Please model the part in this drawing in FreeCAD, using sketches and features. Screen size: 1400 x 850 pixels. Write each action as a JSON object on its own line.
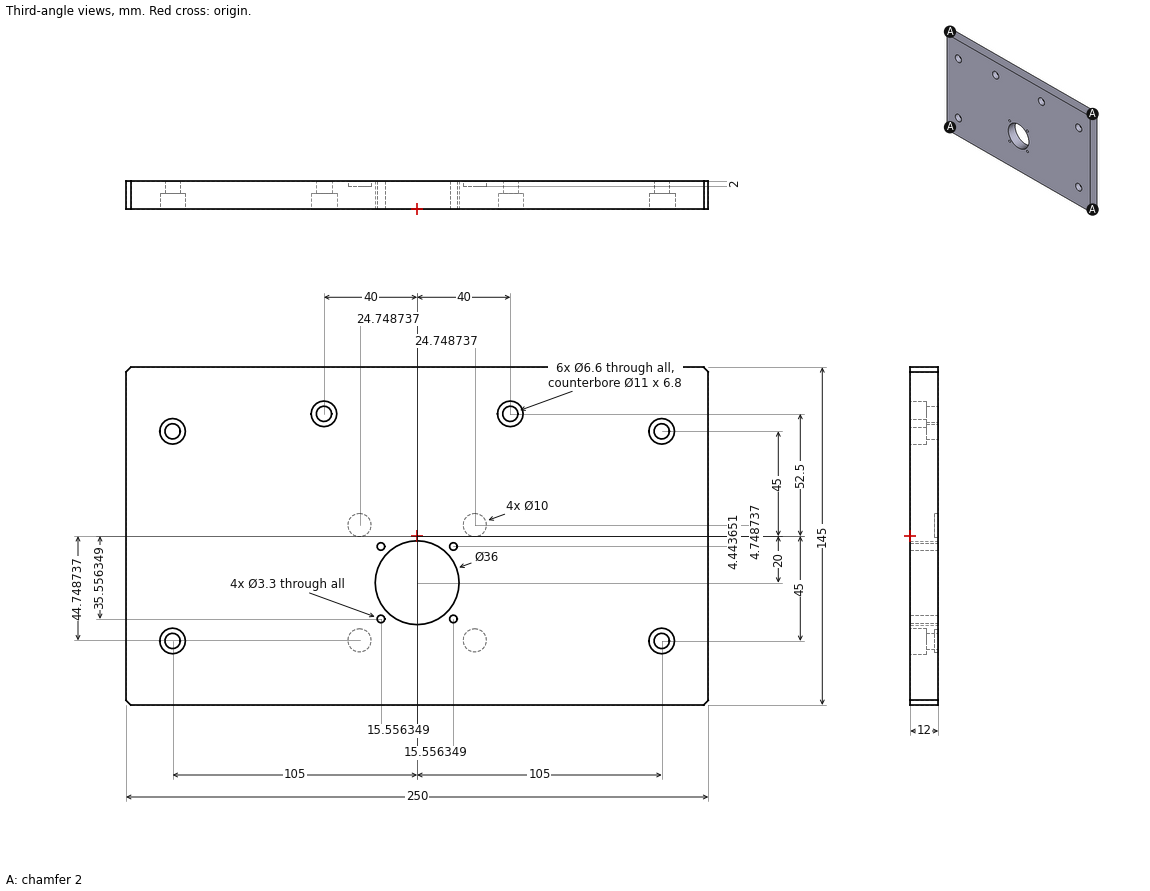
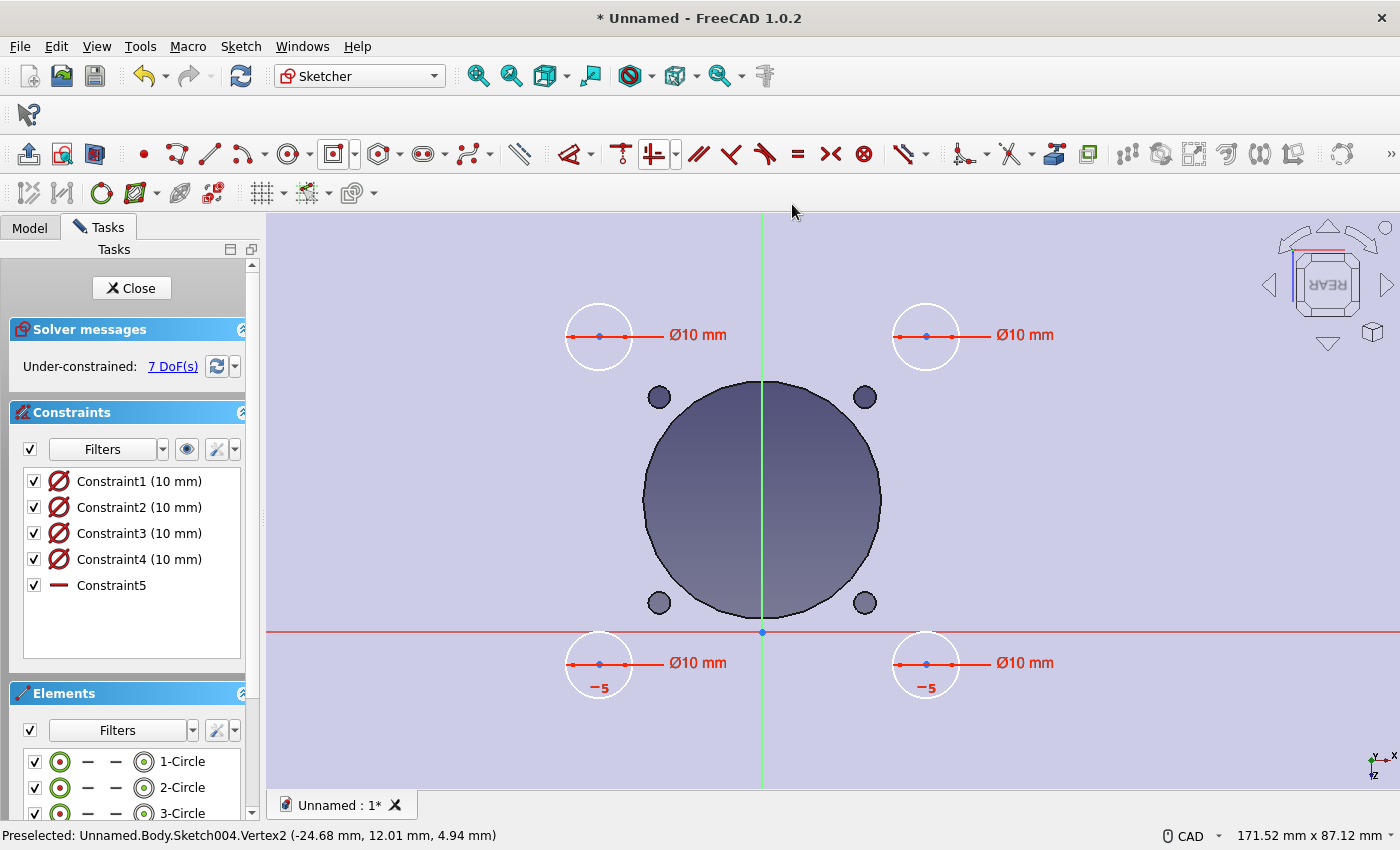
{"action": "left_click", "coordinate": [599, 665]}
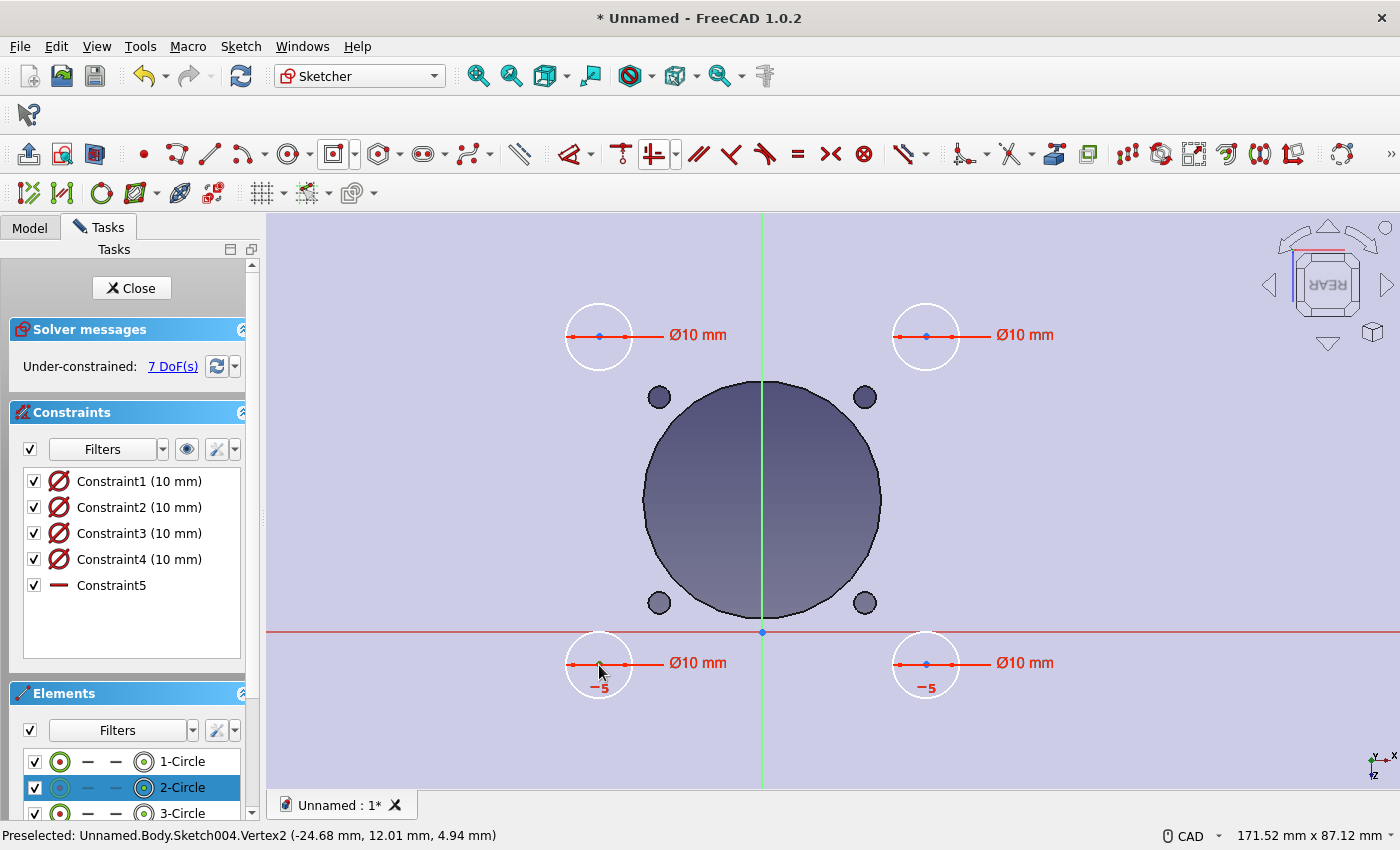
{"action": "left_click", "coordinate": [599, 337]}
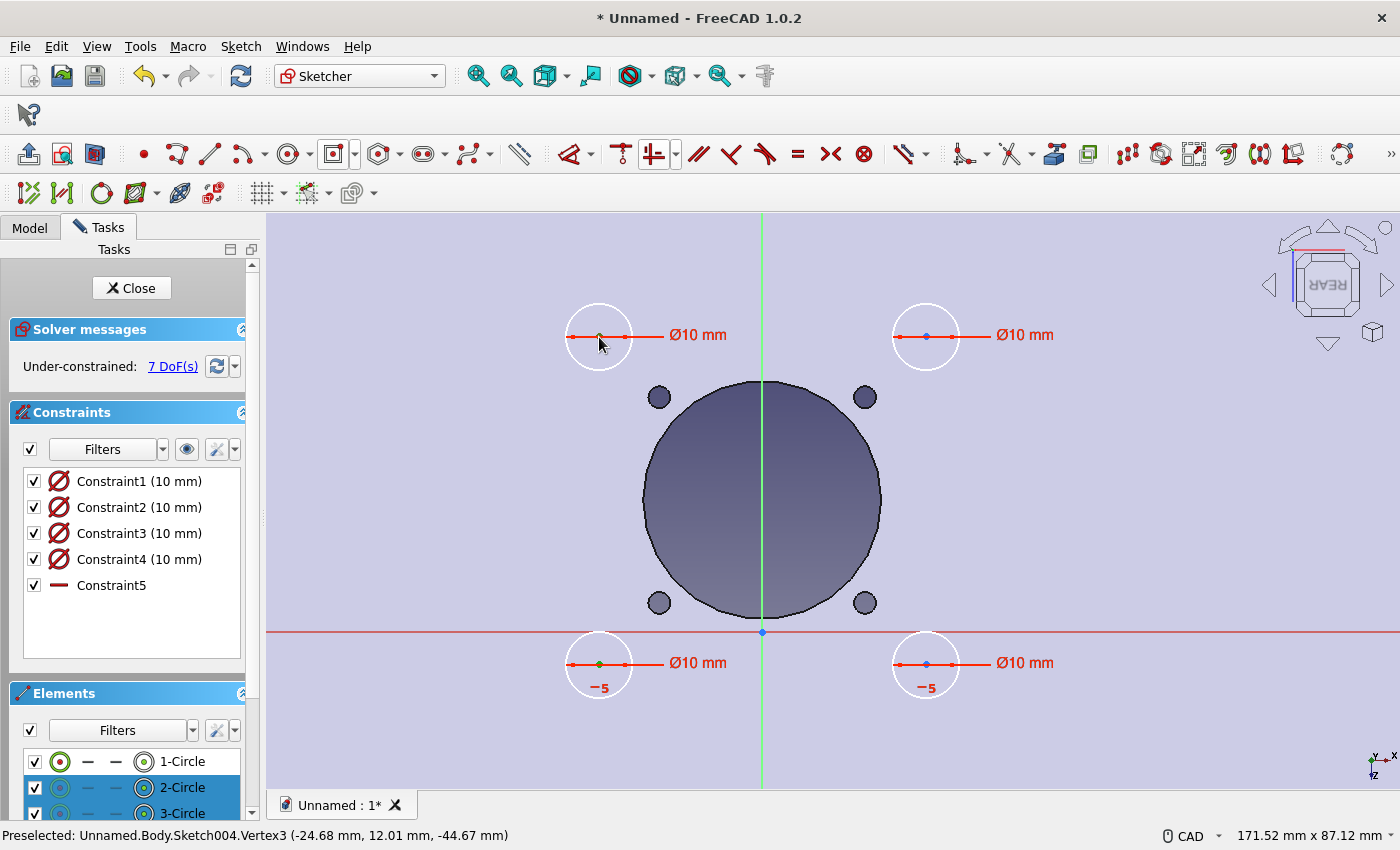
{"action": "left_click", "coordinate": [676, 154]}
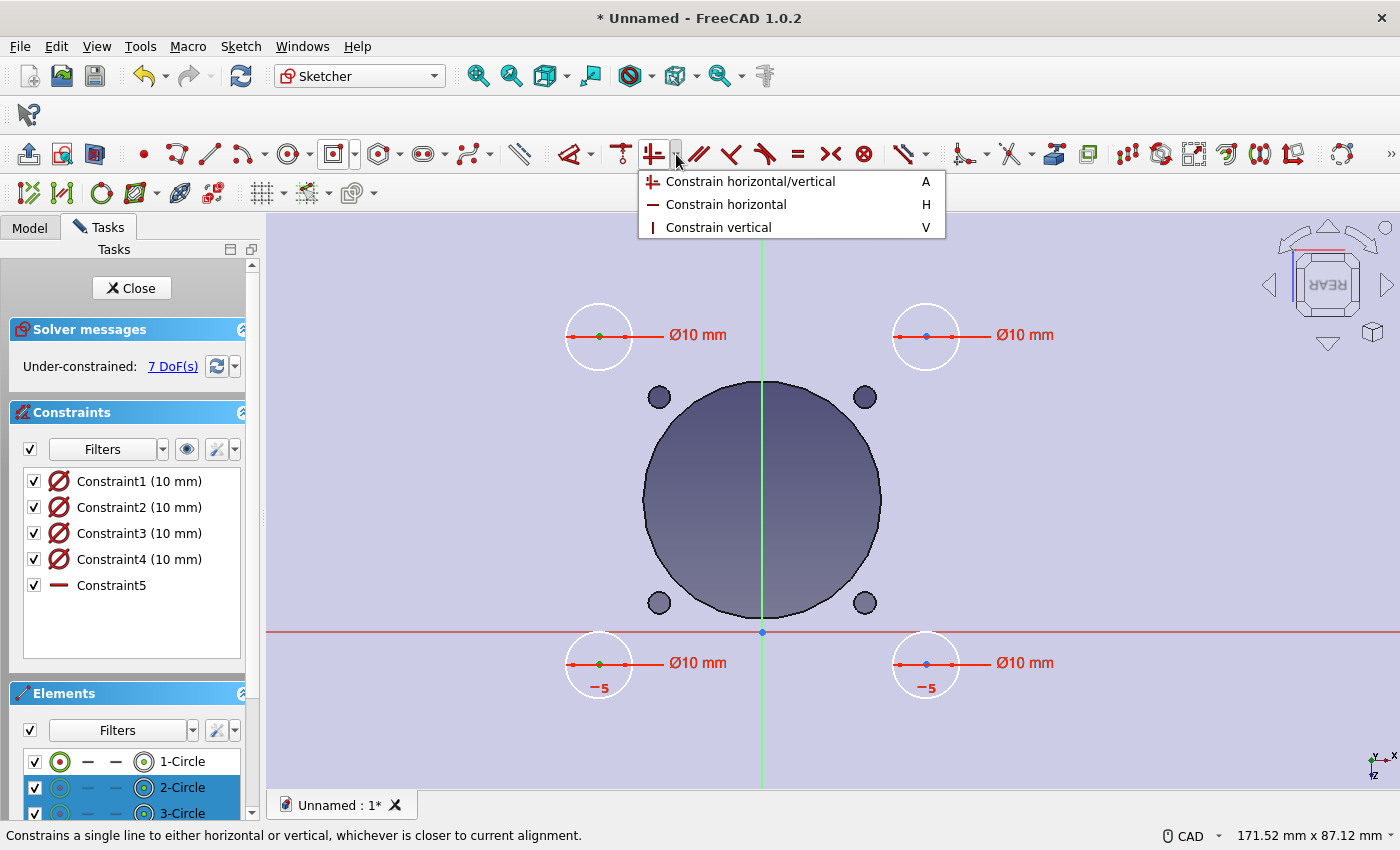
{"action": "left_click", "coordinate": [792, 228]}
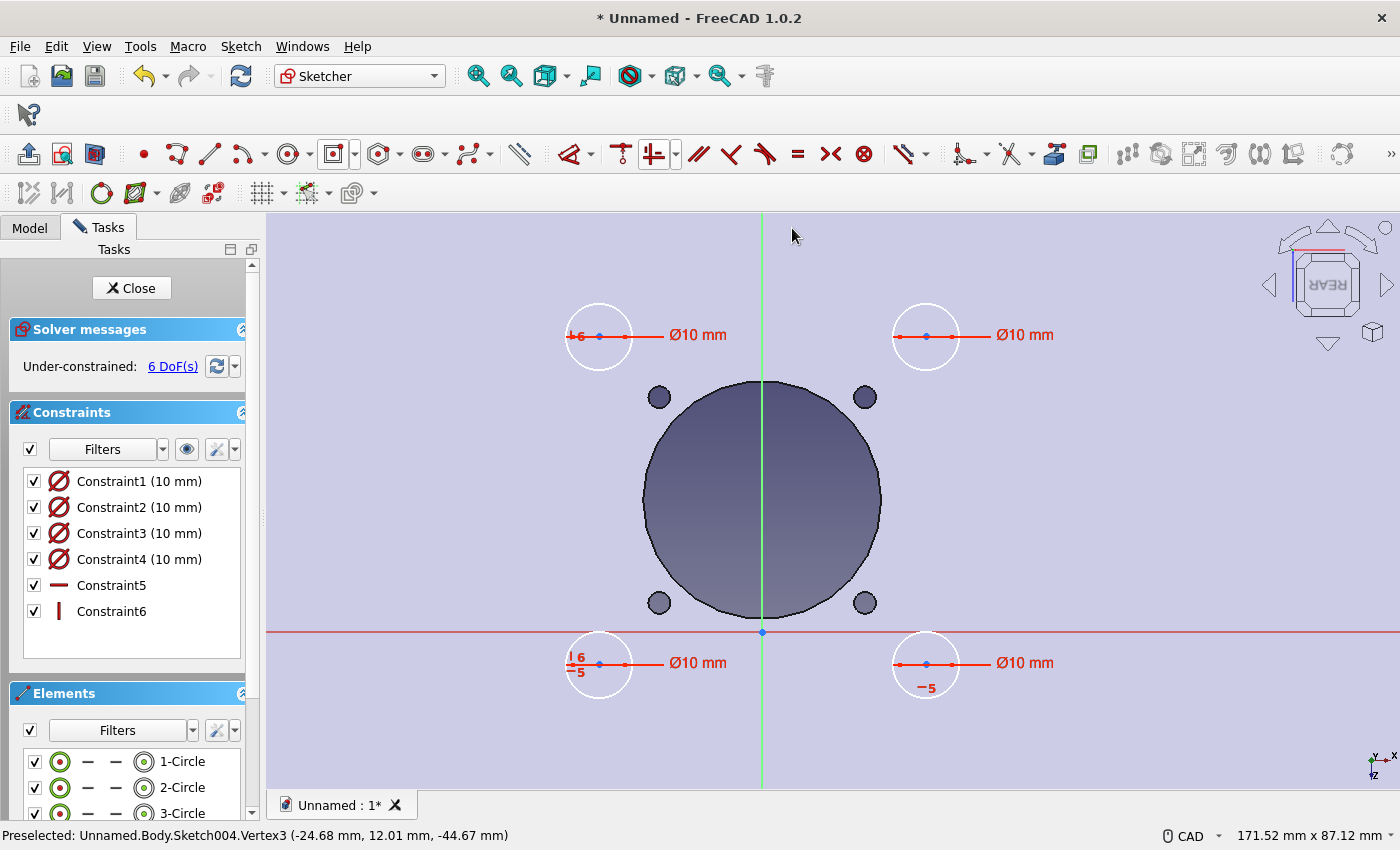
{"action": "left_click", "coordinate": [926, 665]}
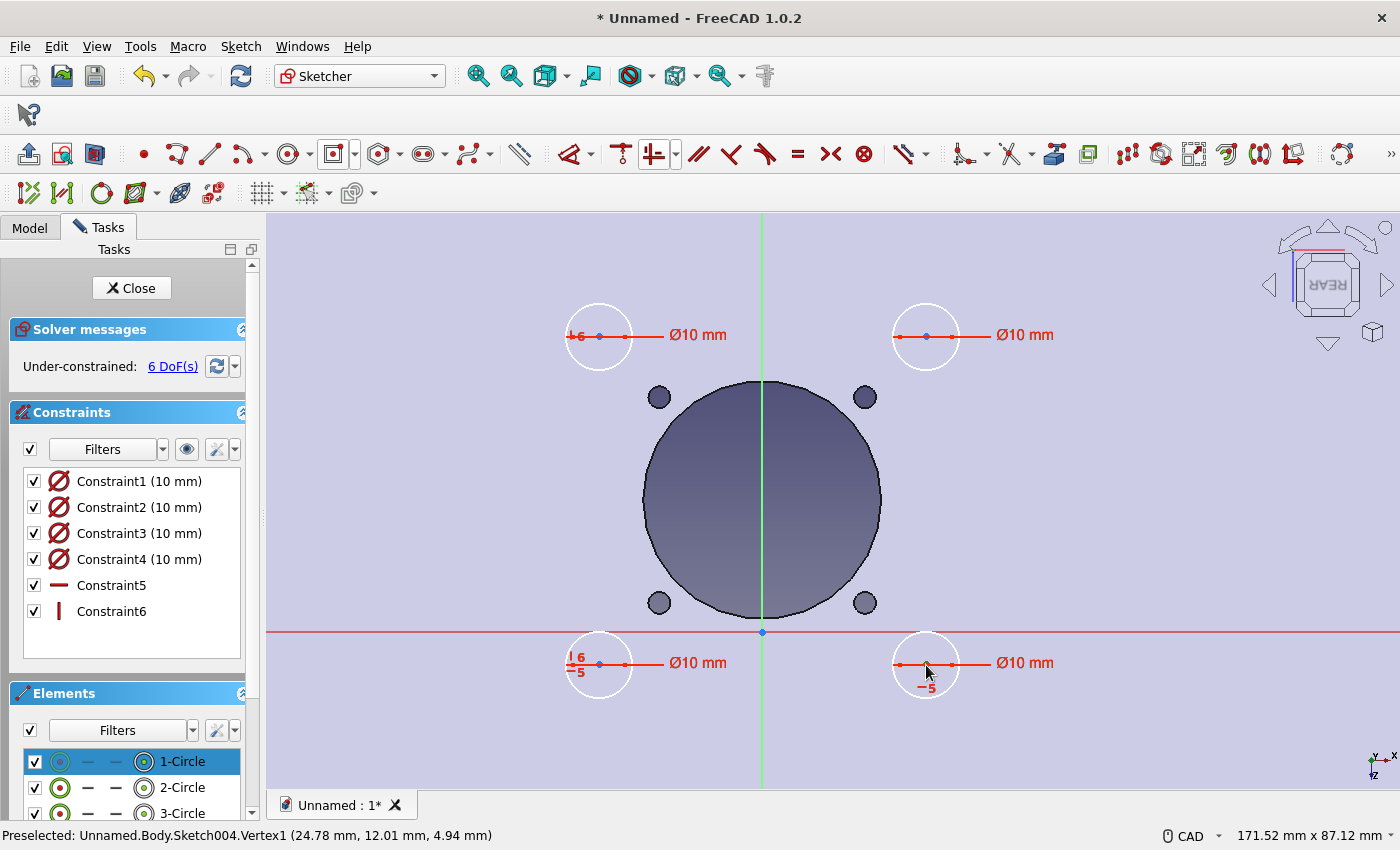
{"action": "left_click", "coordinate": [926, 337]}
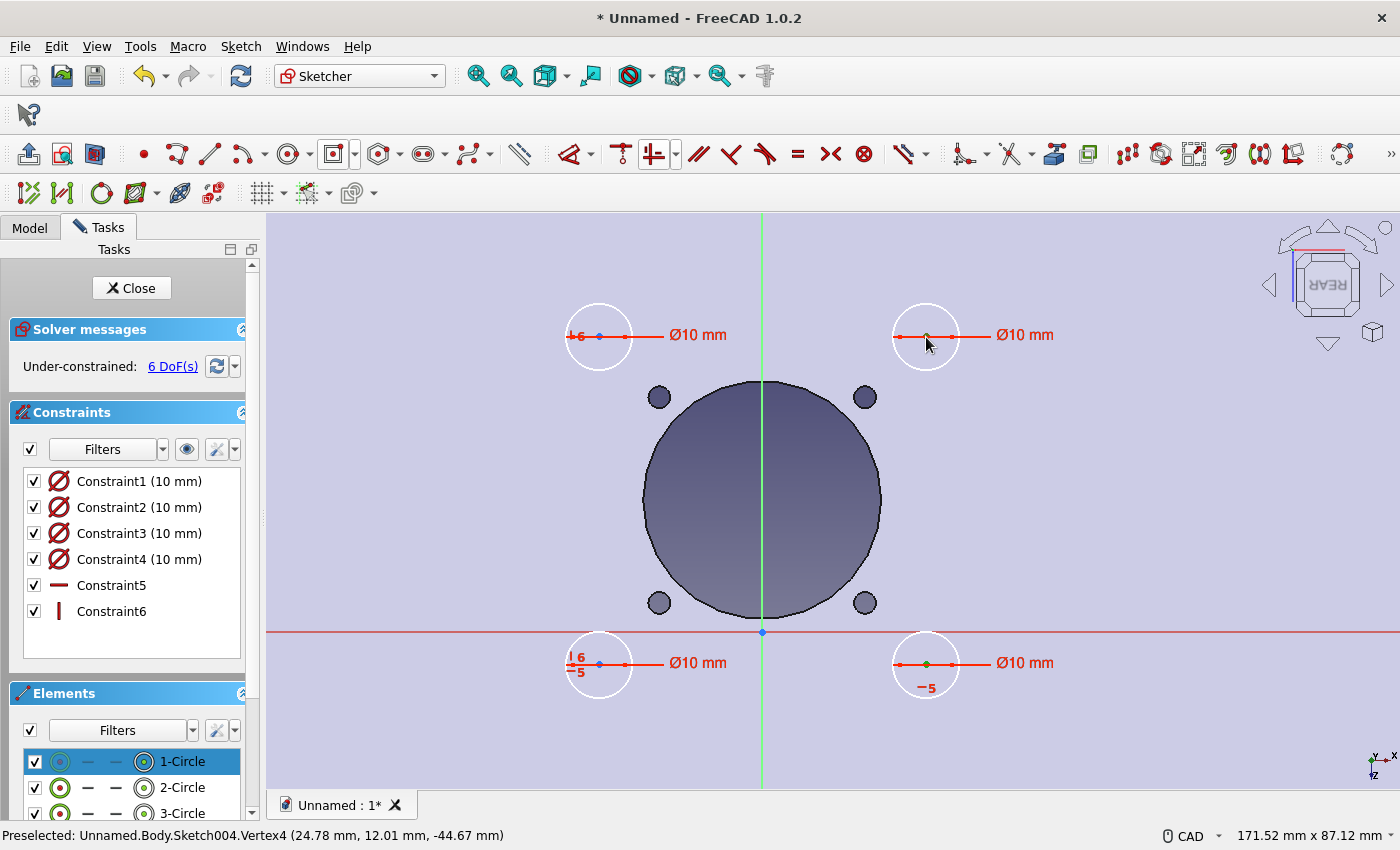
{"action": "key", "text": "v"}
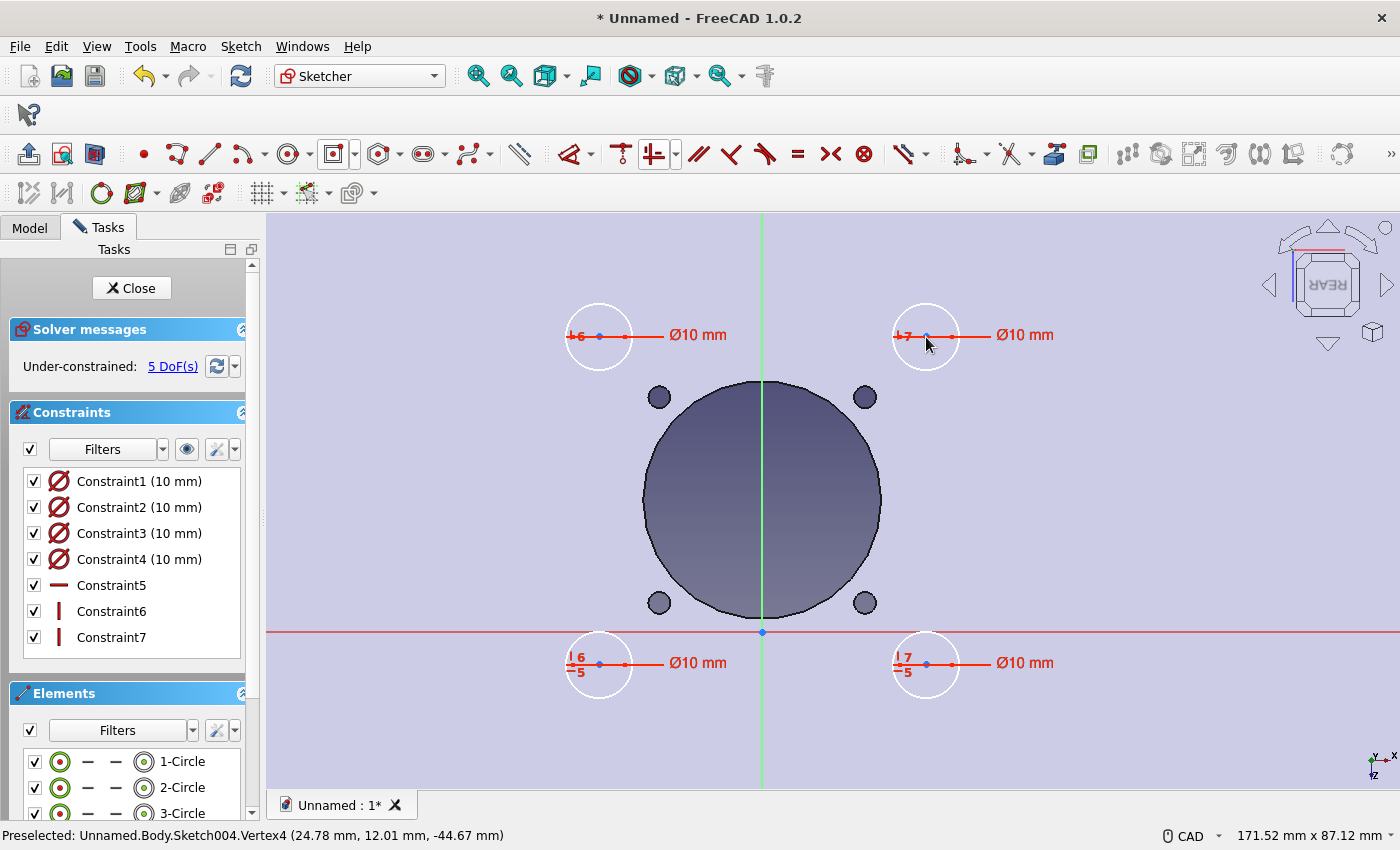
{"action": "left_click", "coordinate": [599, 337]}